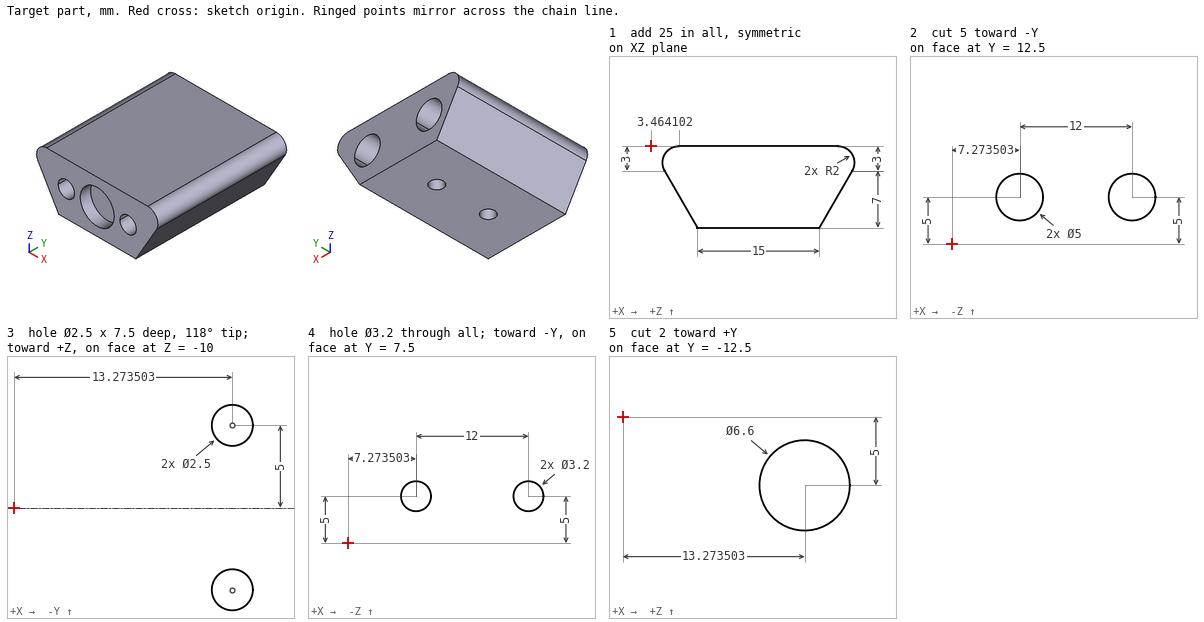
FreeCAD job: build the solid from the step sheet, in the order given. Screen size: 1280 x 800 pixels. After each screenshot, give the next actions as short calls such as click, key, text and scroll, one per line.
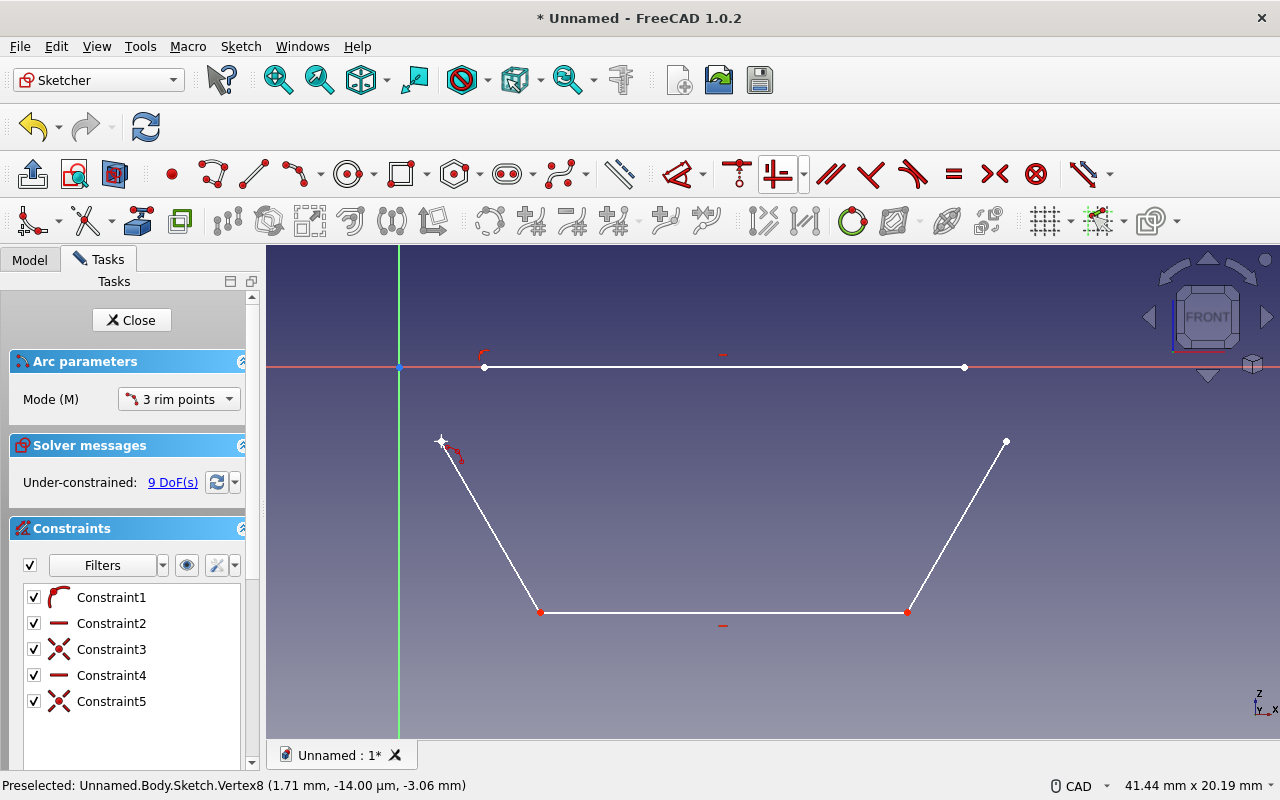
click(964, 367)
click(1006, 442)
click(1006, 392)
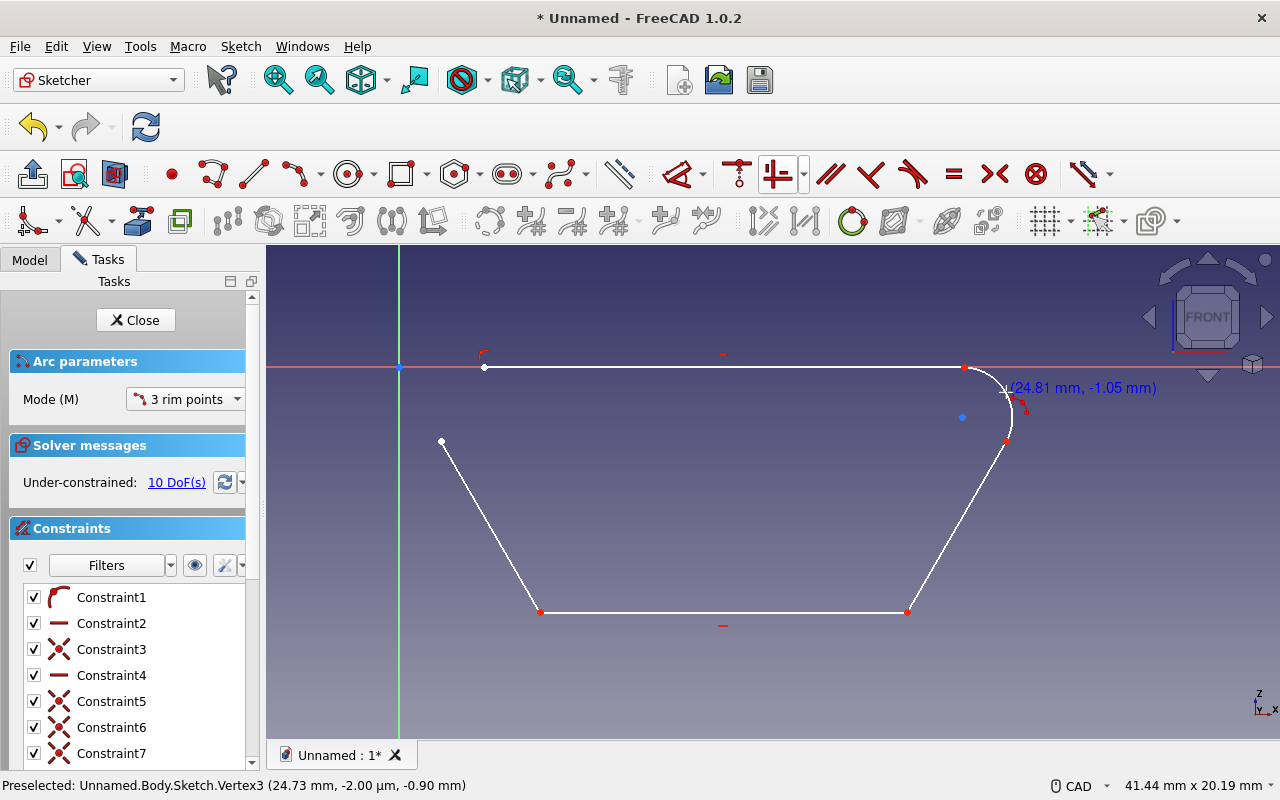
click(441, 442)
click(484, 367)
click(441, 392)
key(Escape)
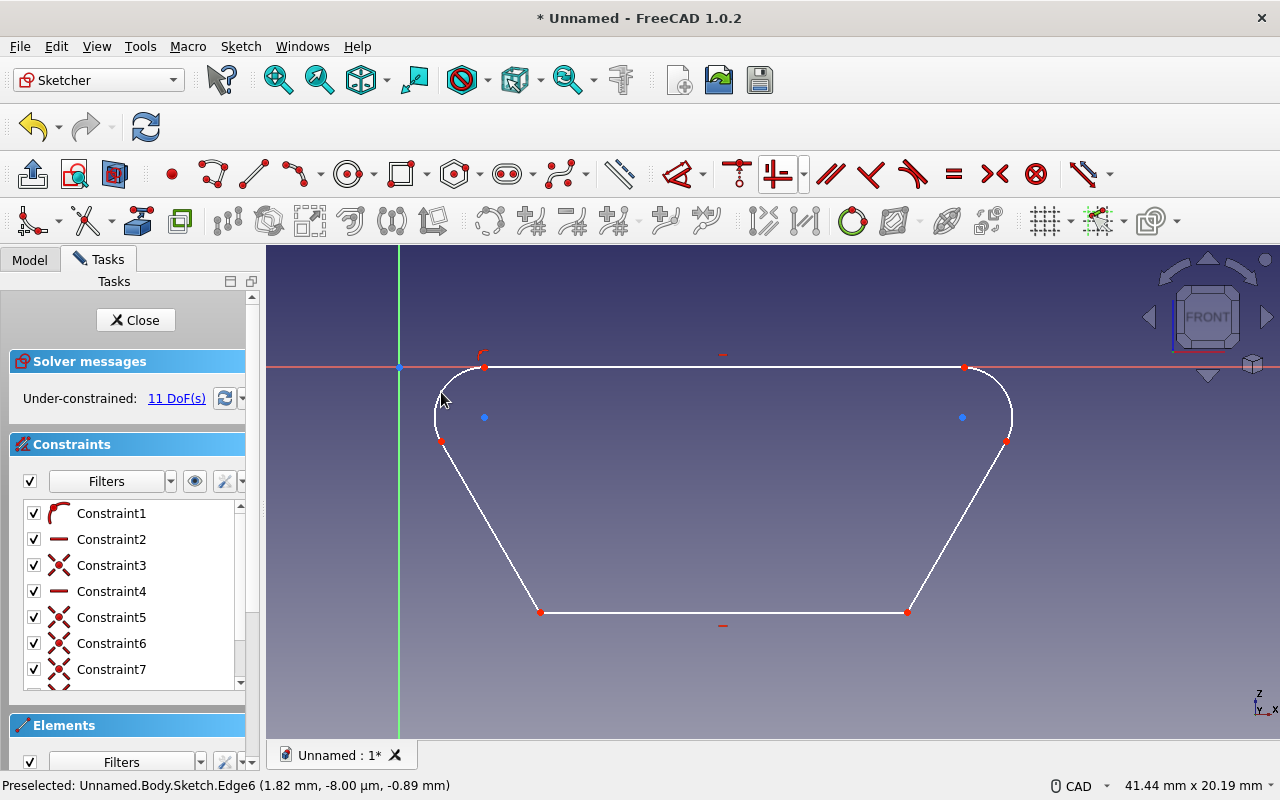
click(628, 367)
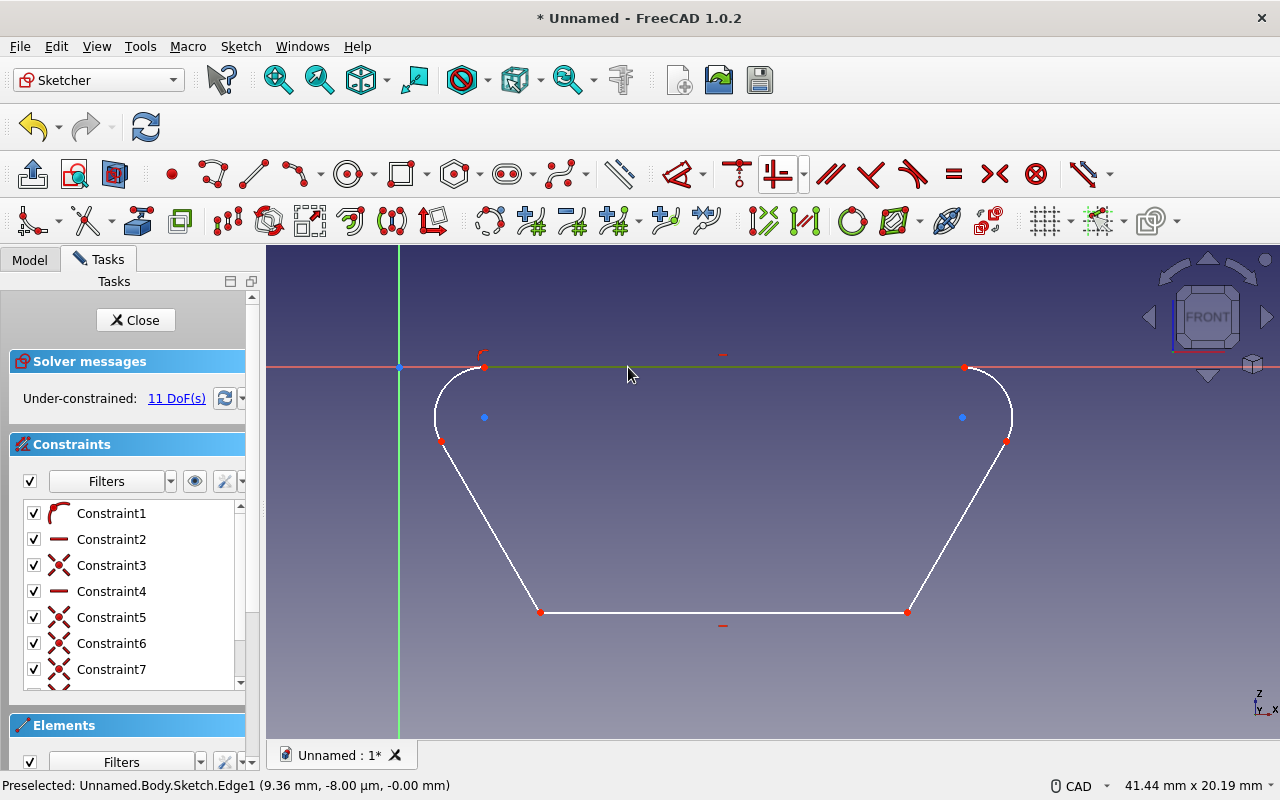
click(1012, 412)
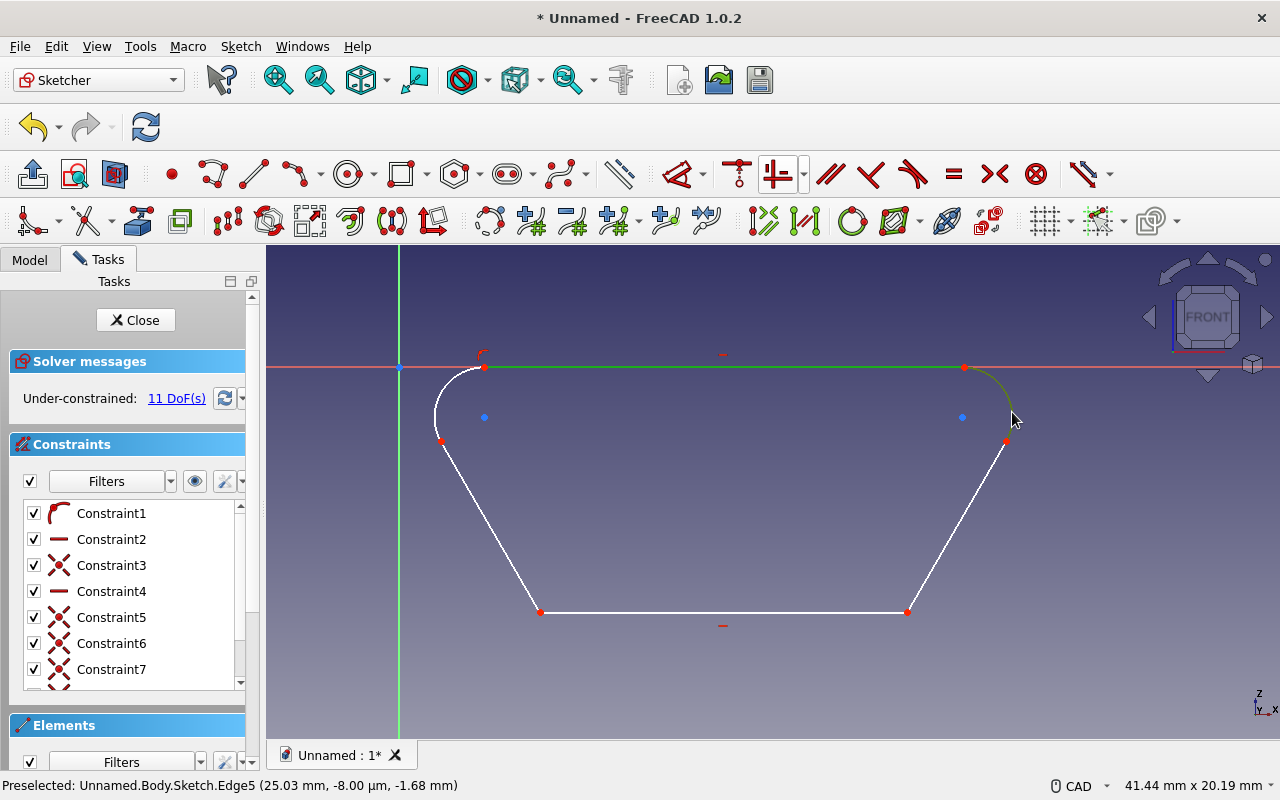
click(913, 174)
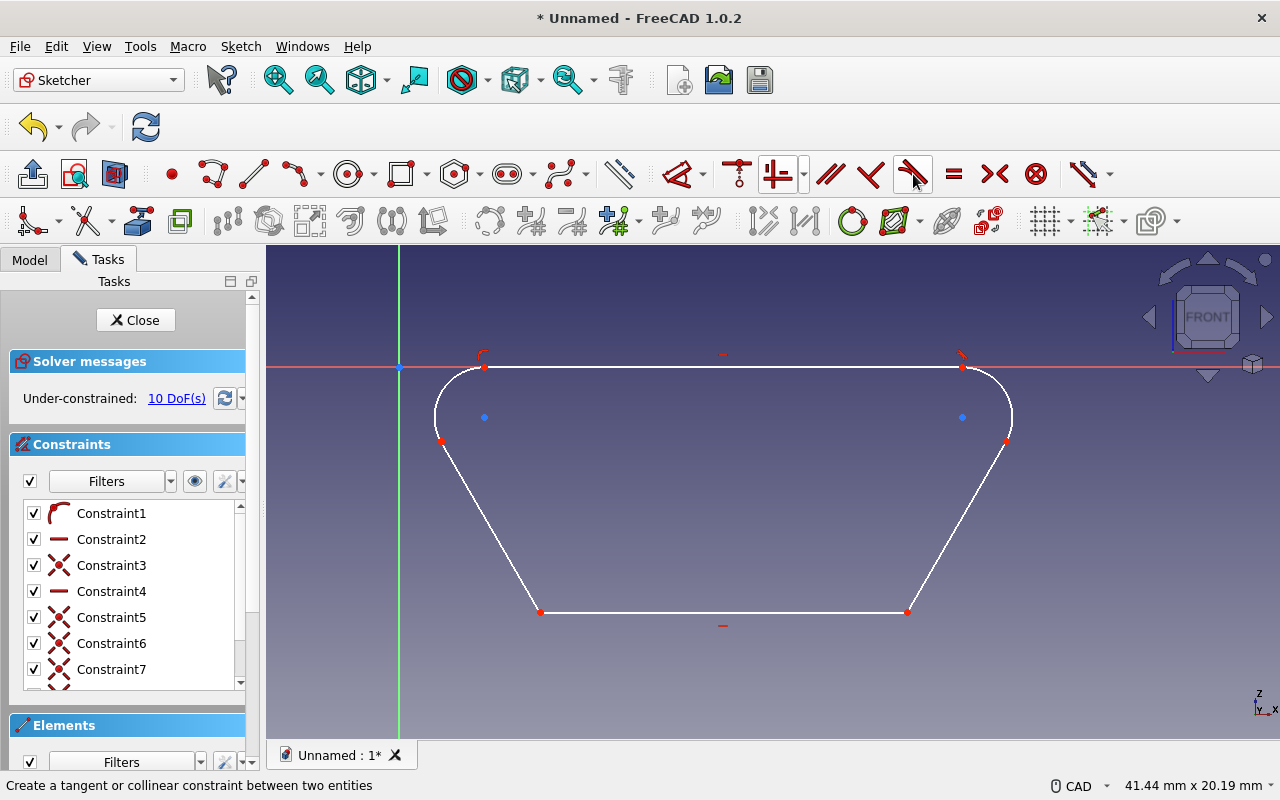
click(627, 367)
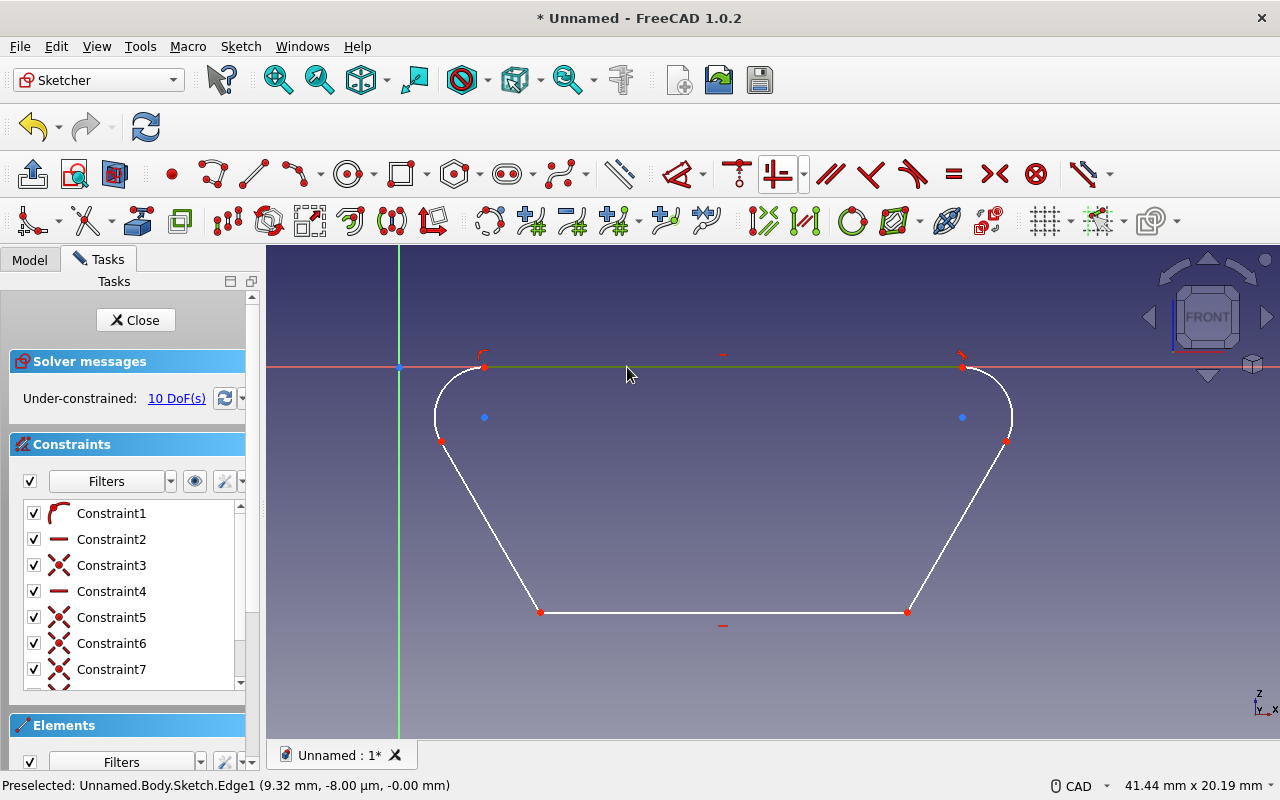
scroll(455, 377, up, 2)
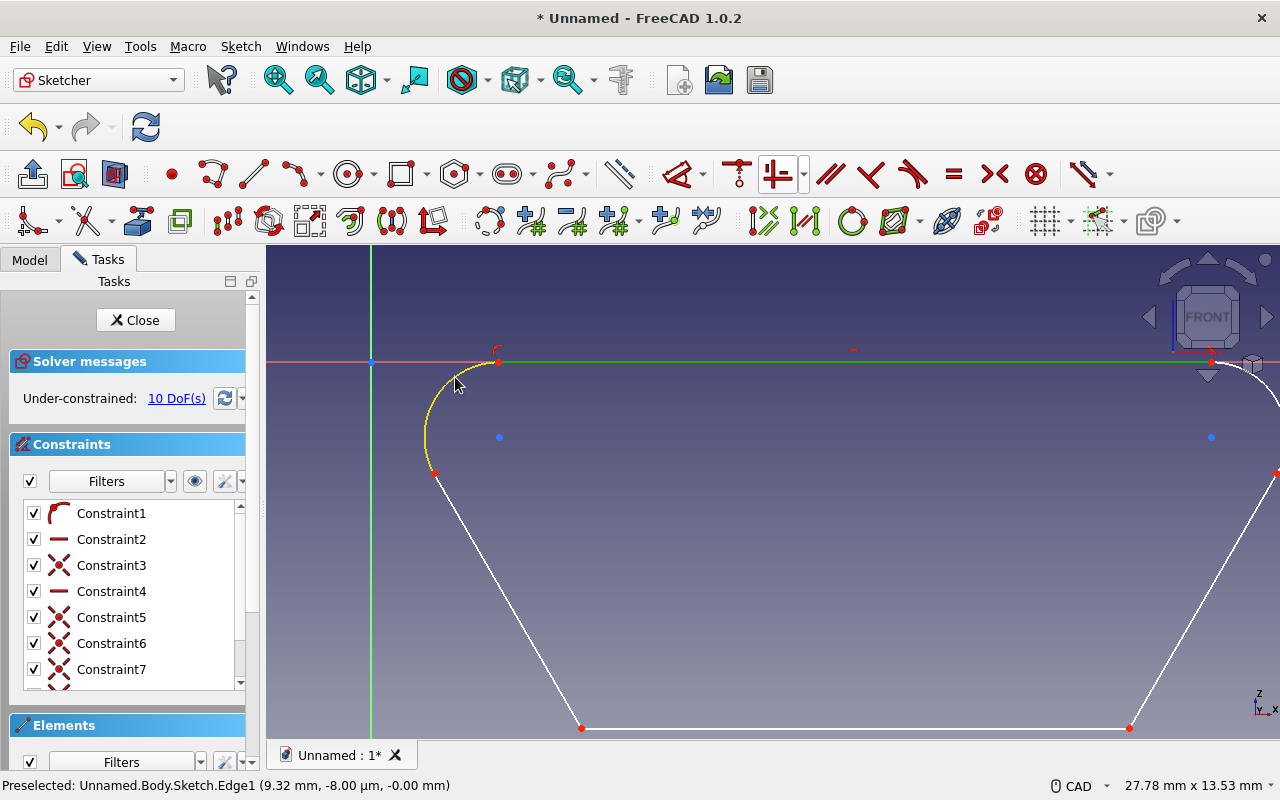
click(455, 377)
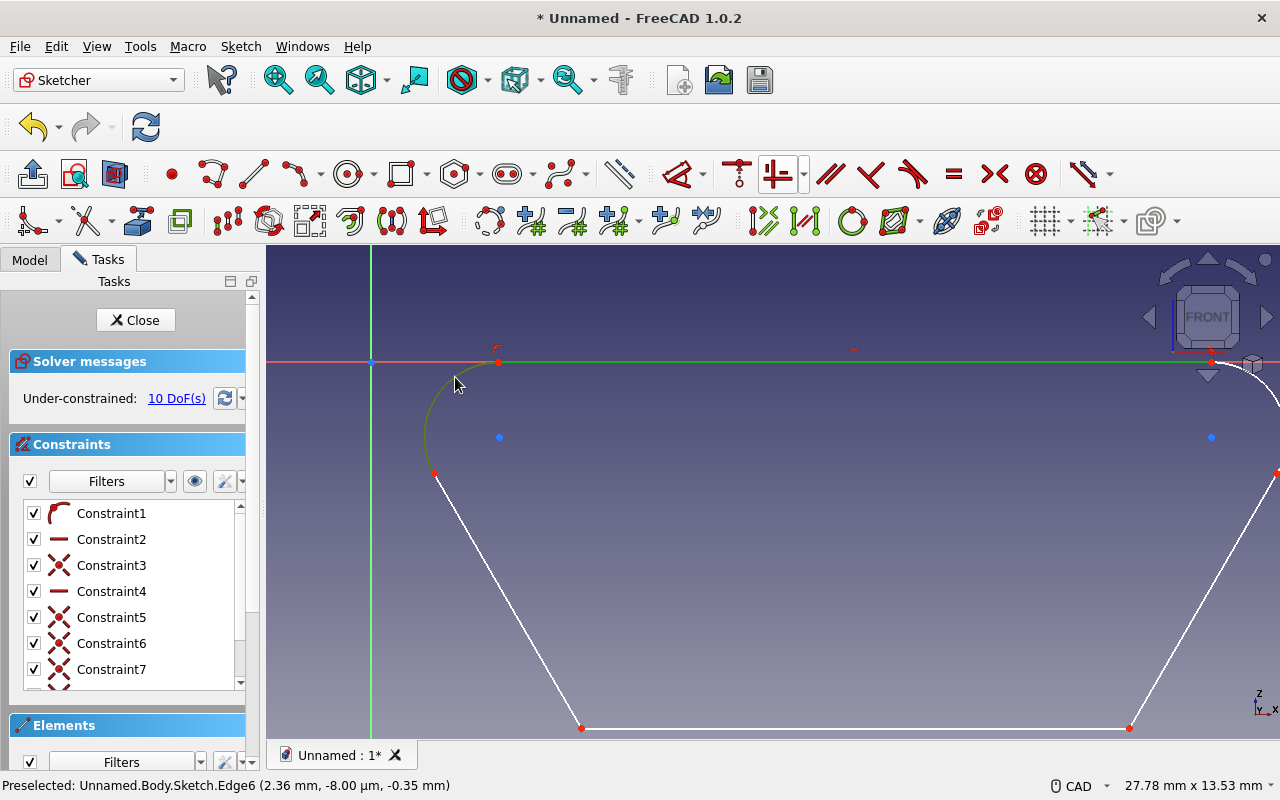
click(913, 174)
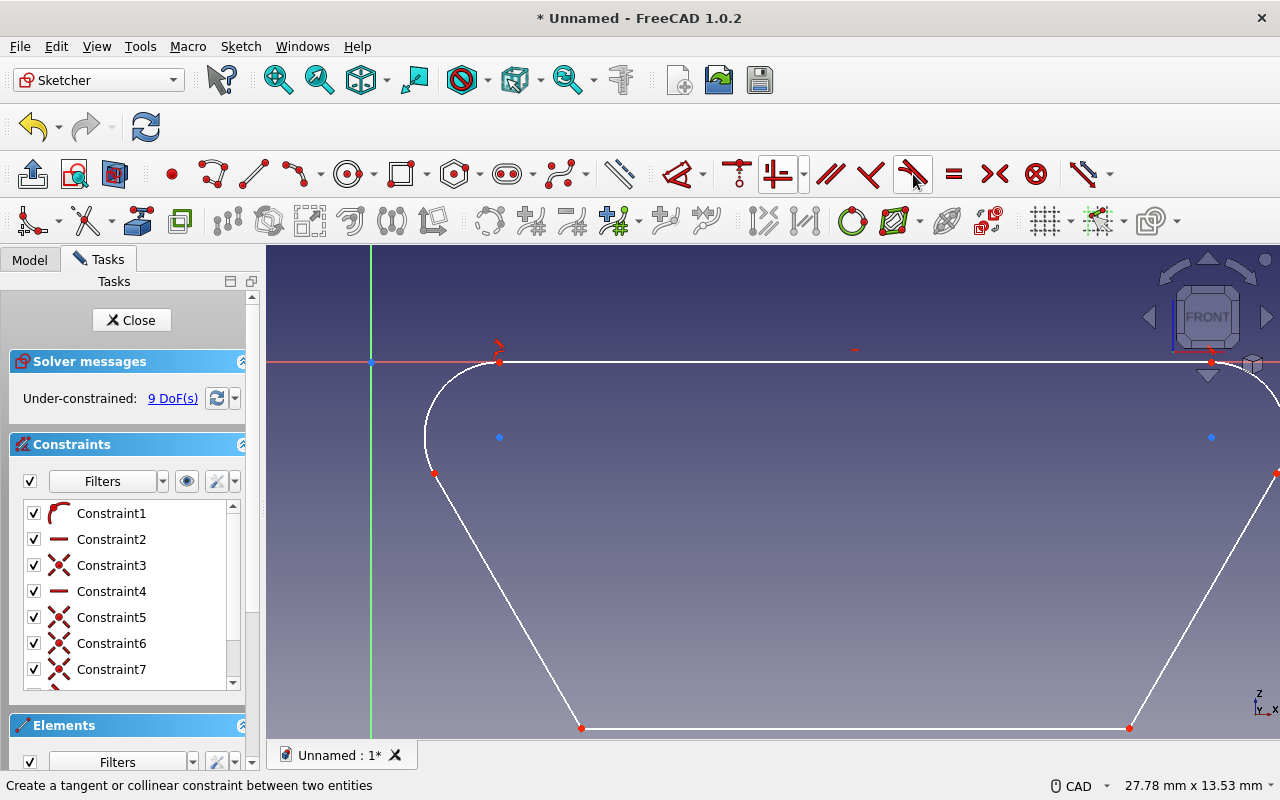
scroll(461, 385, down, 2)